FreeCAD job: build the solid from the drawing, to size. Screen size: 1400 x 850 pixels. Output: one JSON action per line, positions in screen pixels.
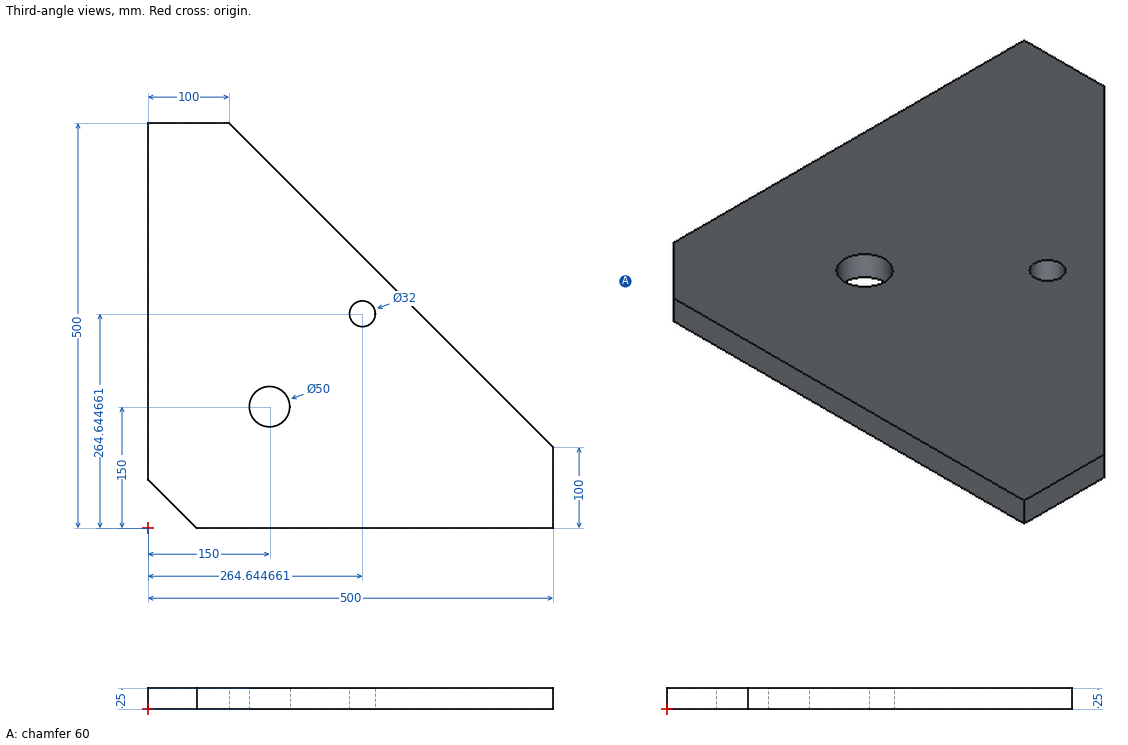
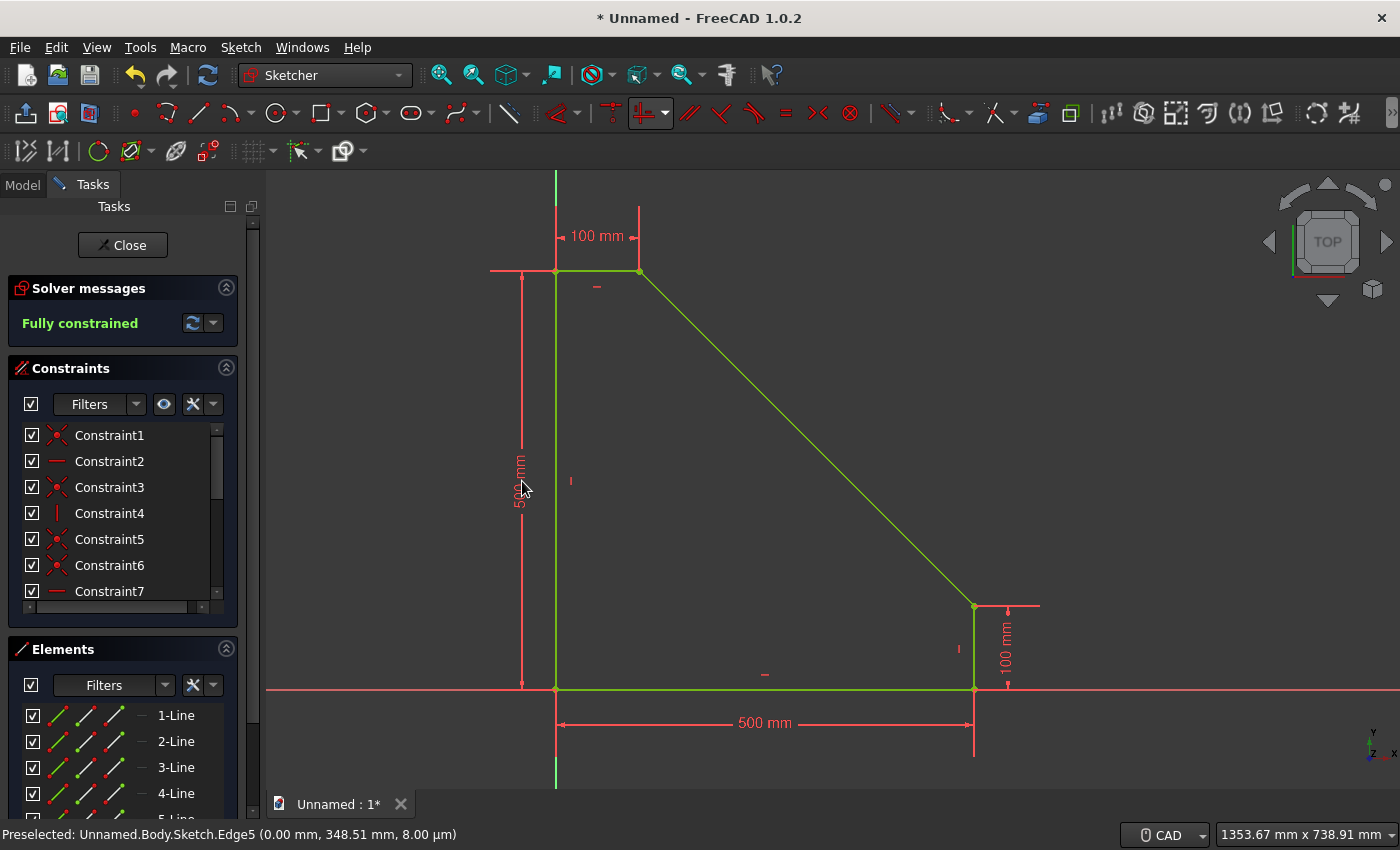
{"action": "left_click", "coordinate": [123, 245]}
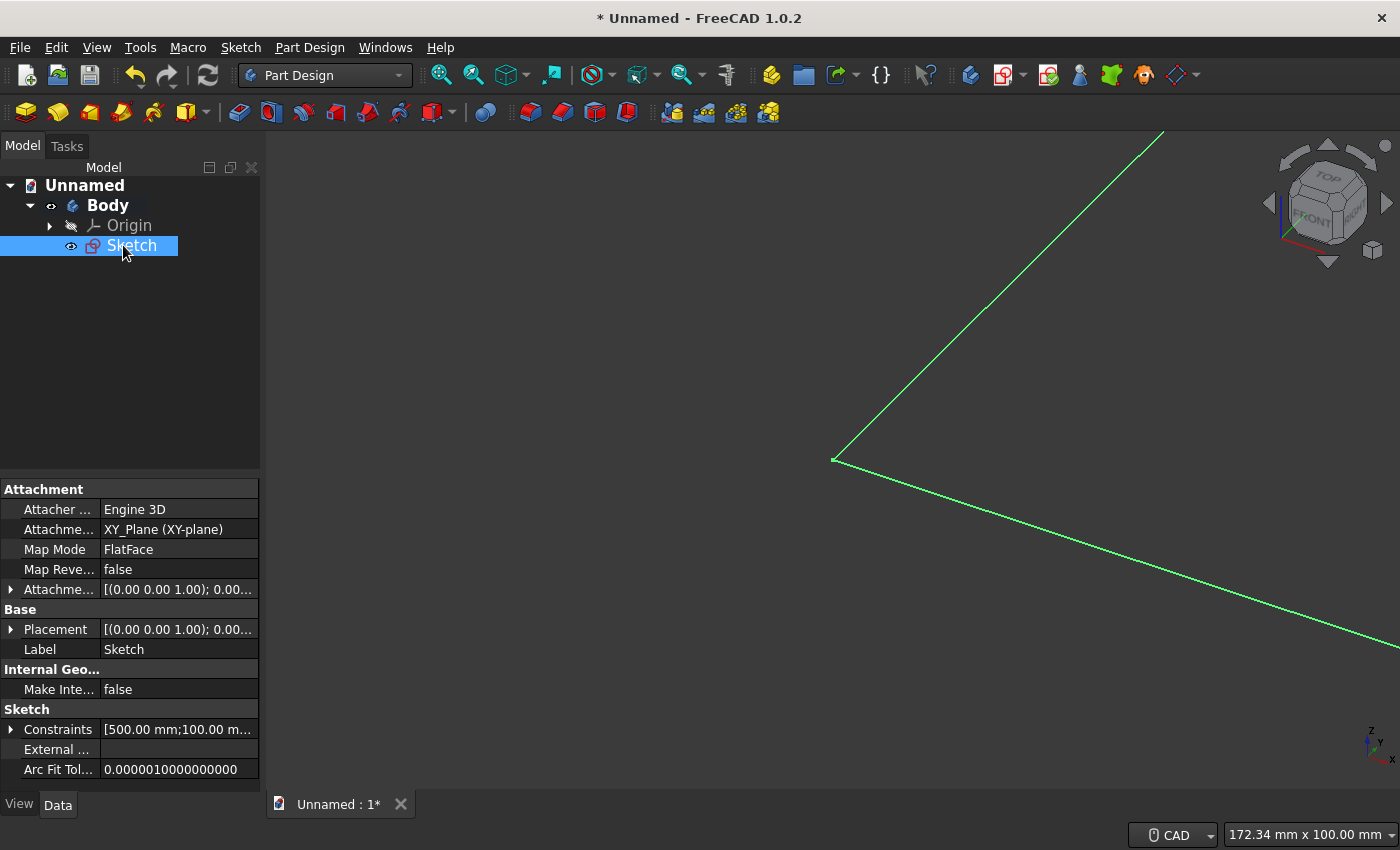
{"action": "left_click", "coordinate": [26, 112]}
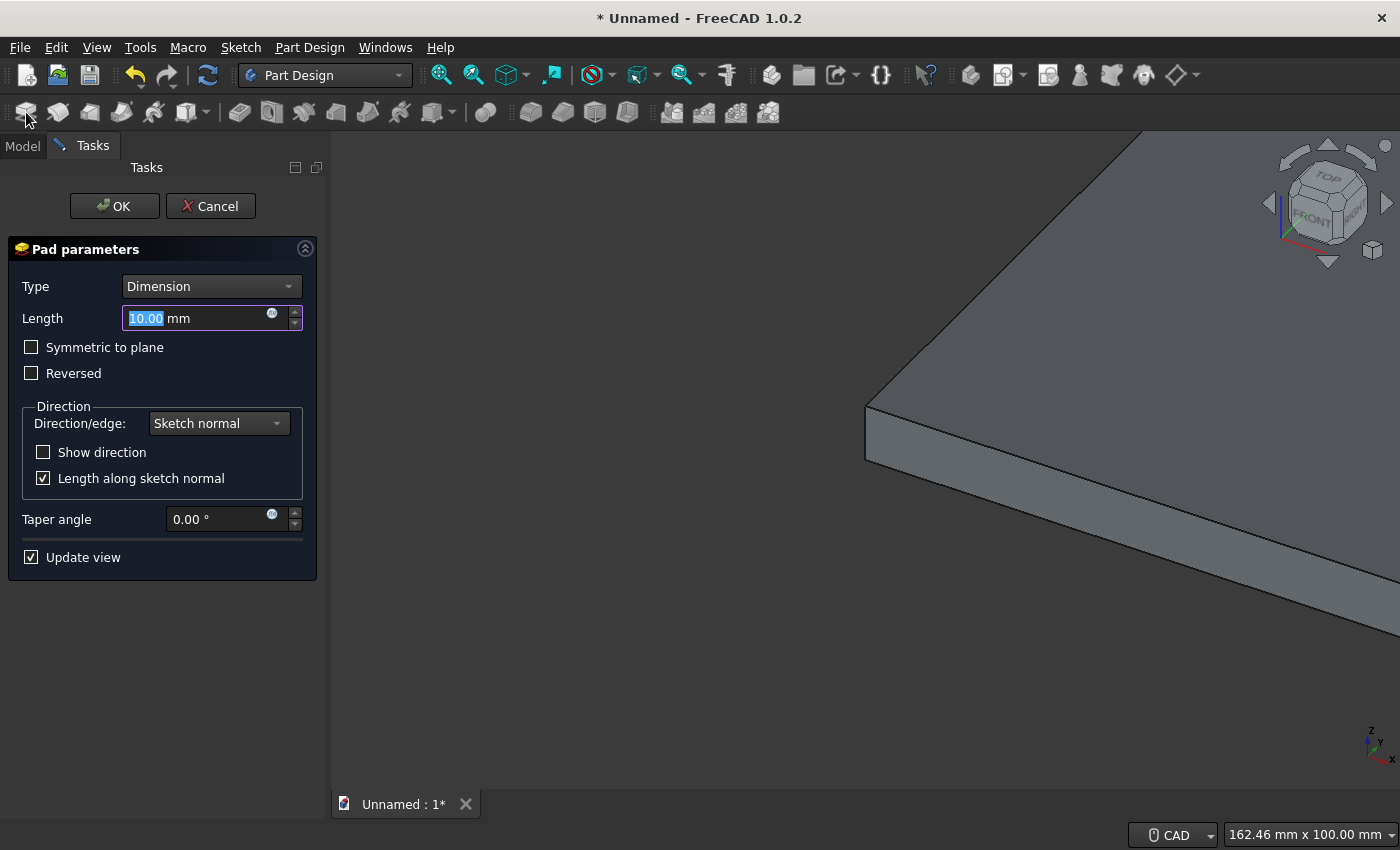
{"action": "type", "text": "25"}
{"action": "key", "text": "Tab"}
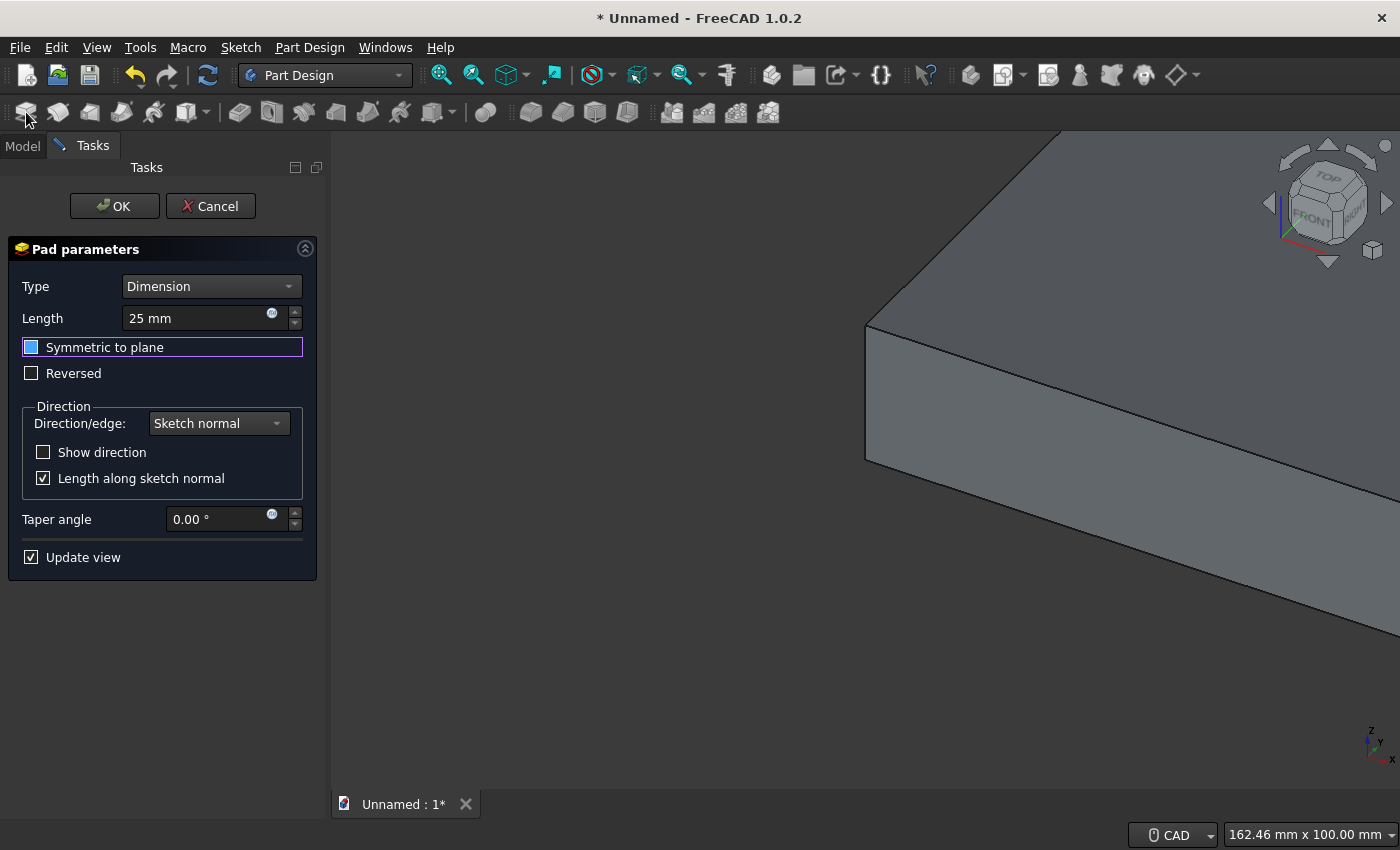
{"action": "left_click", "coordinate": [115, 206]}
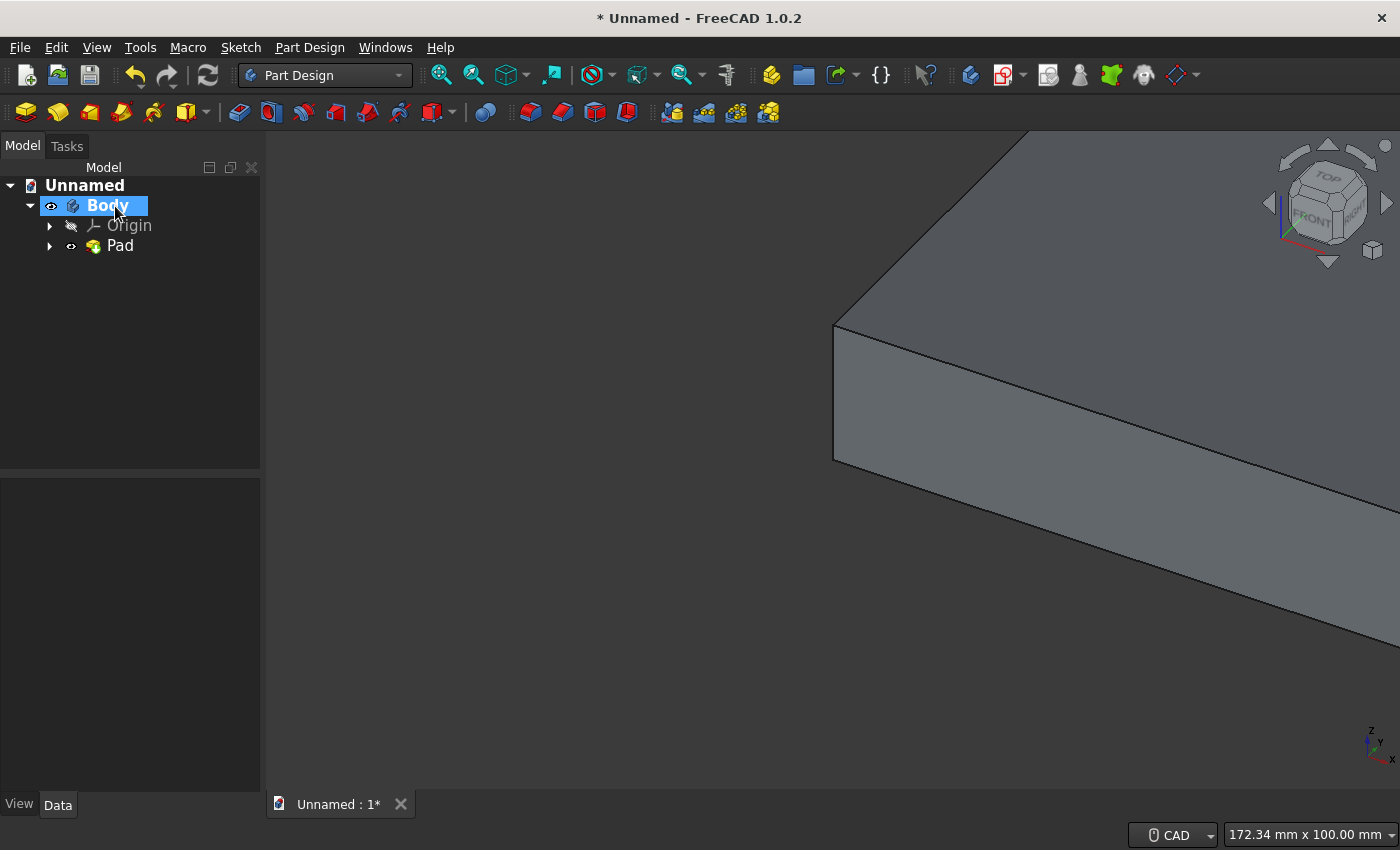
{"action": "left_click", "coordinate": [442, 76]}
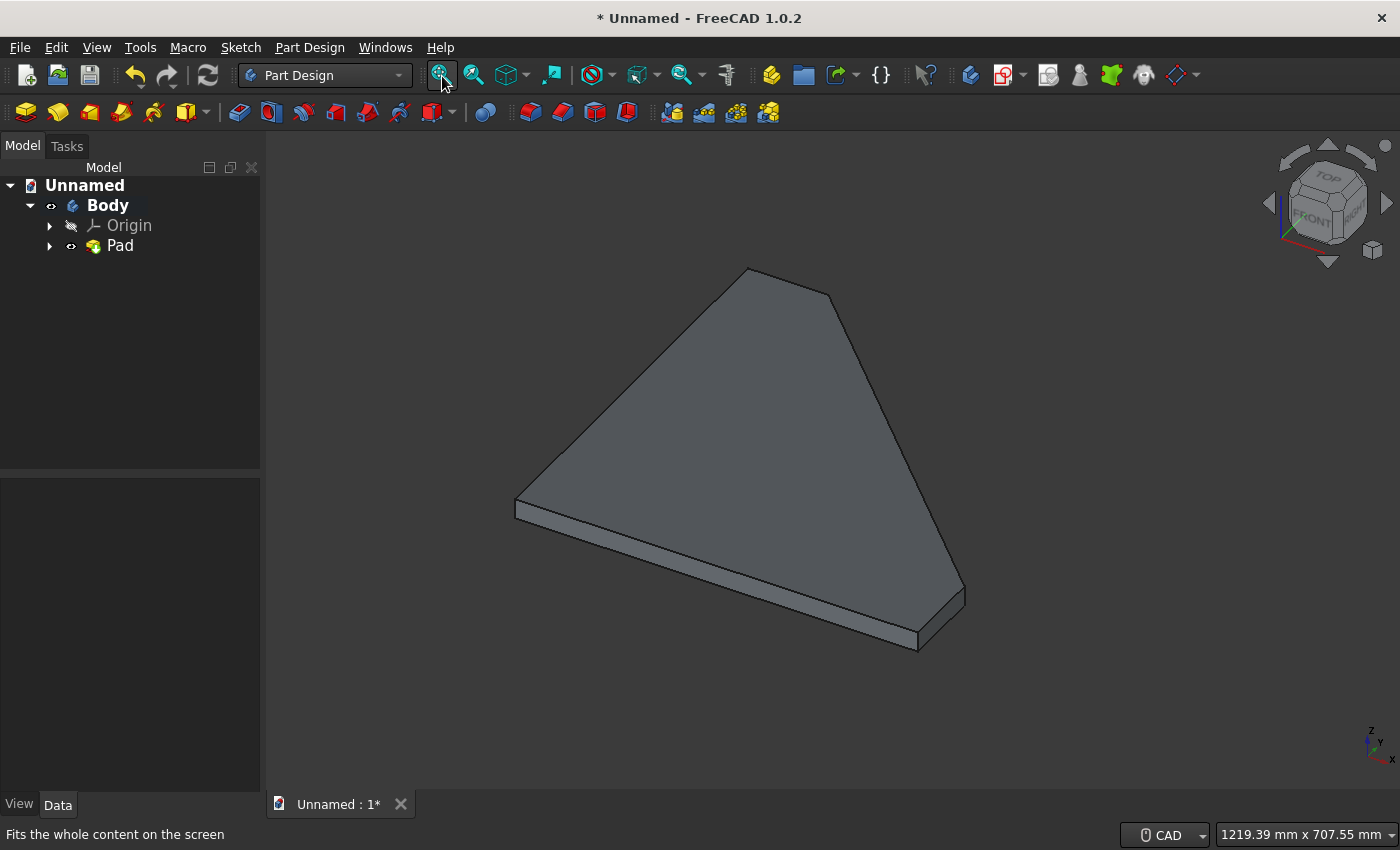
{"action": "left_click", "coordinate": [742, 463]}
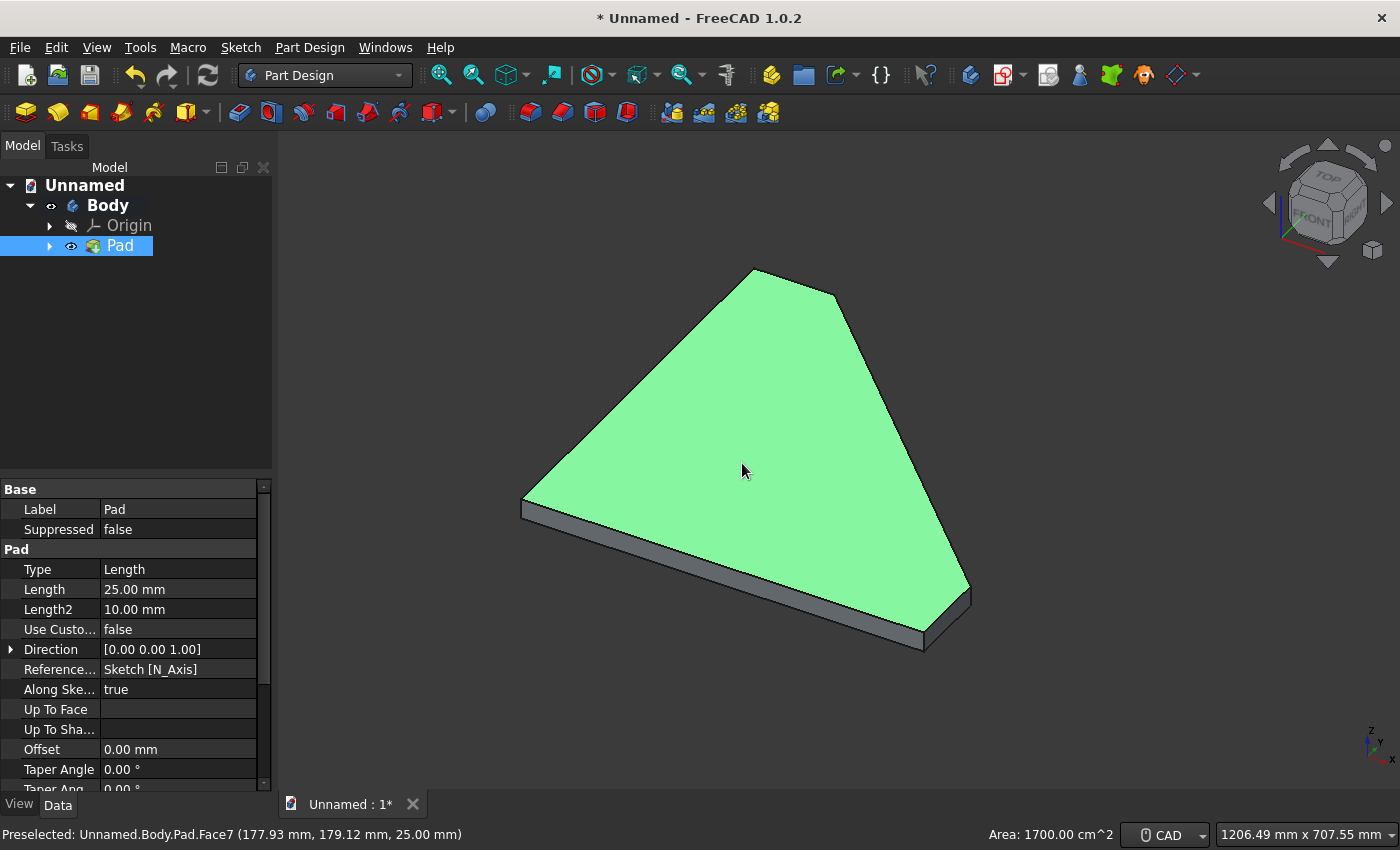
{"action": "left_click", "coordinate": [1004, 76]}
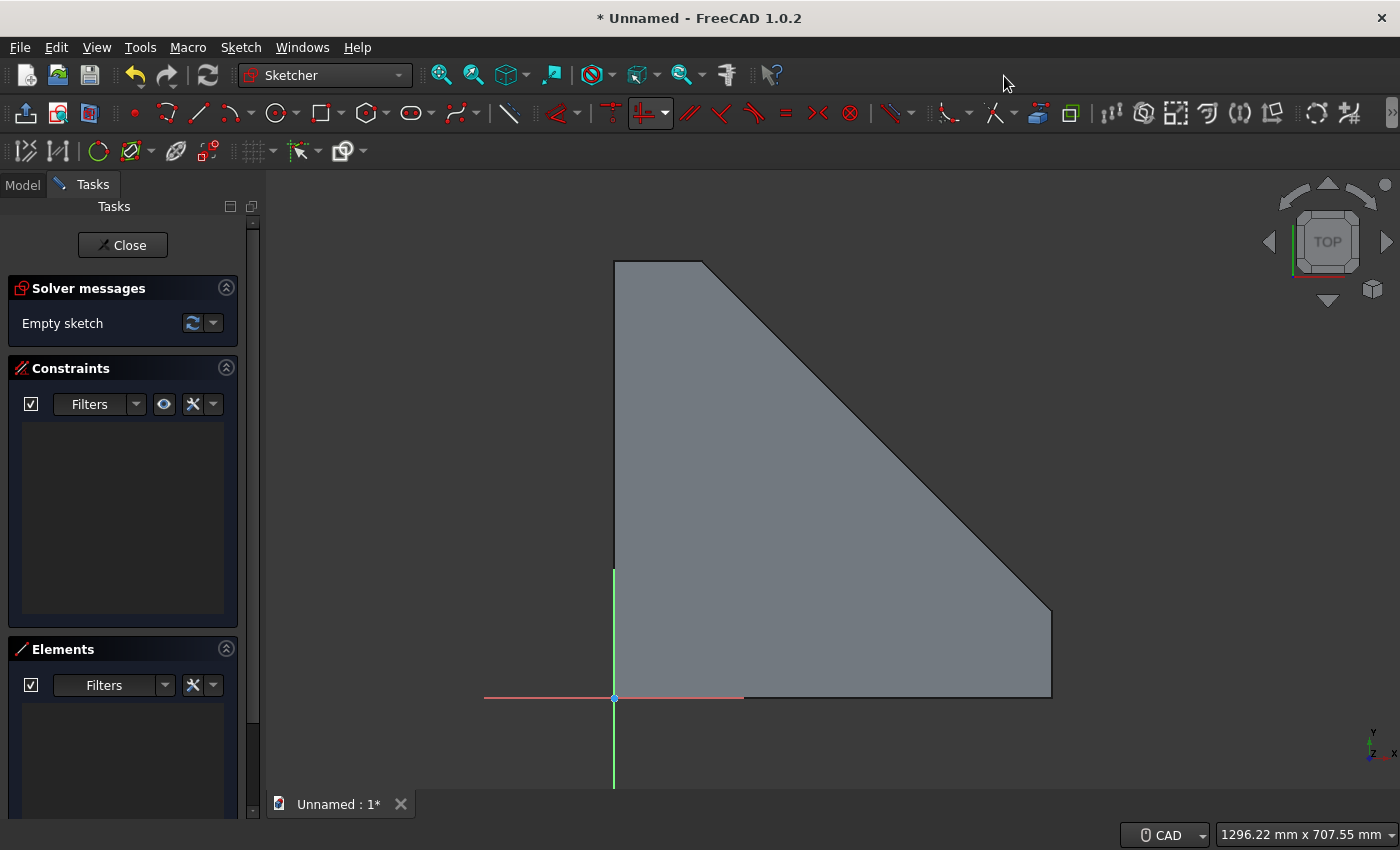
{"action": "scroll", "coordinate": [743, 578], "scroll_direction": "up", "scroll_amount": 11}